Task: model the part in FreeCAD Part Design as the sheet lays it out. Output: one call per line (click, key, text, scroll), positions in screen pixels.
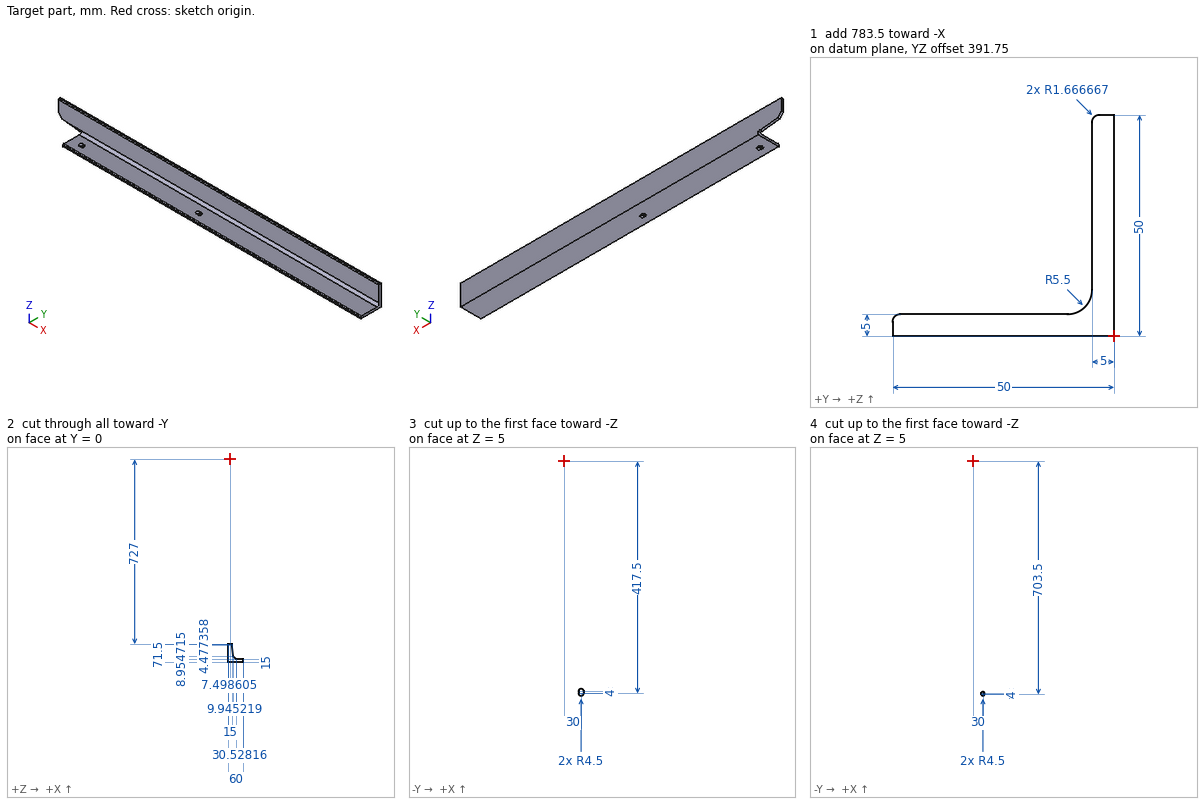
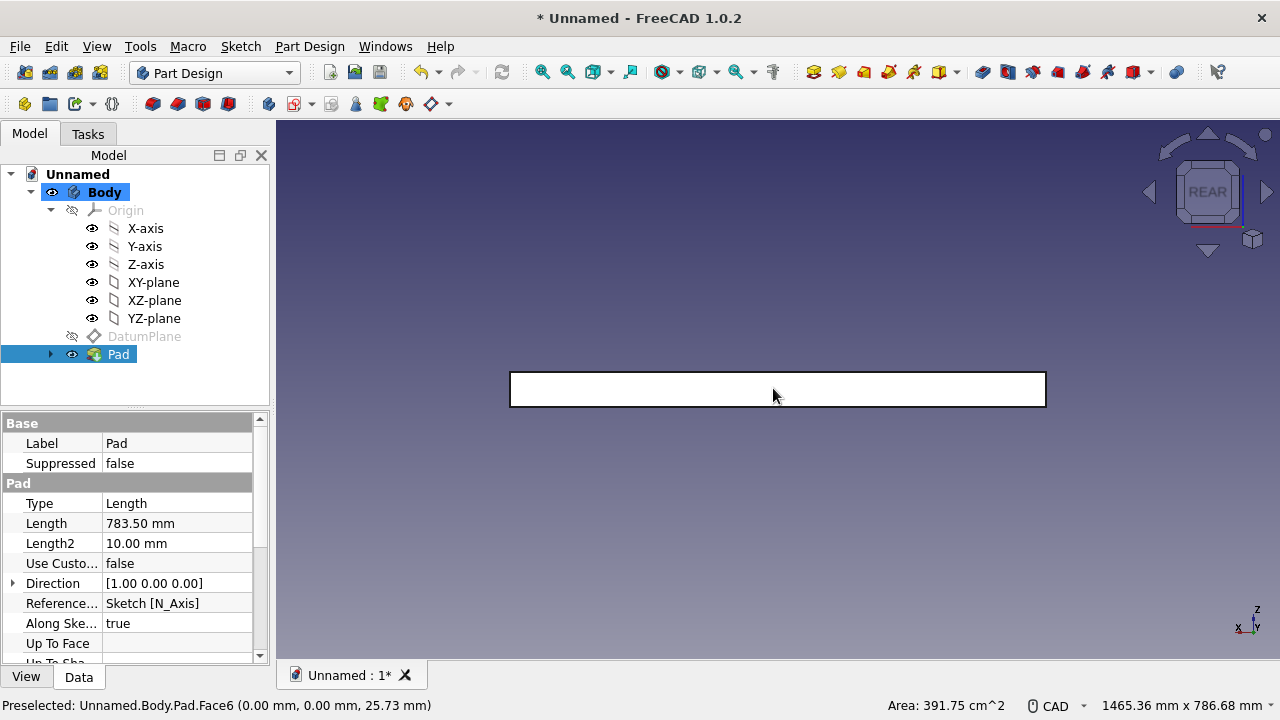
click(294, 104)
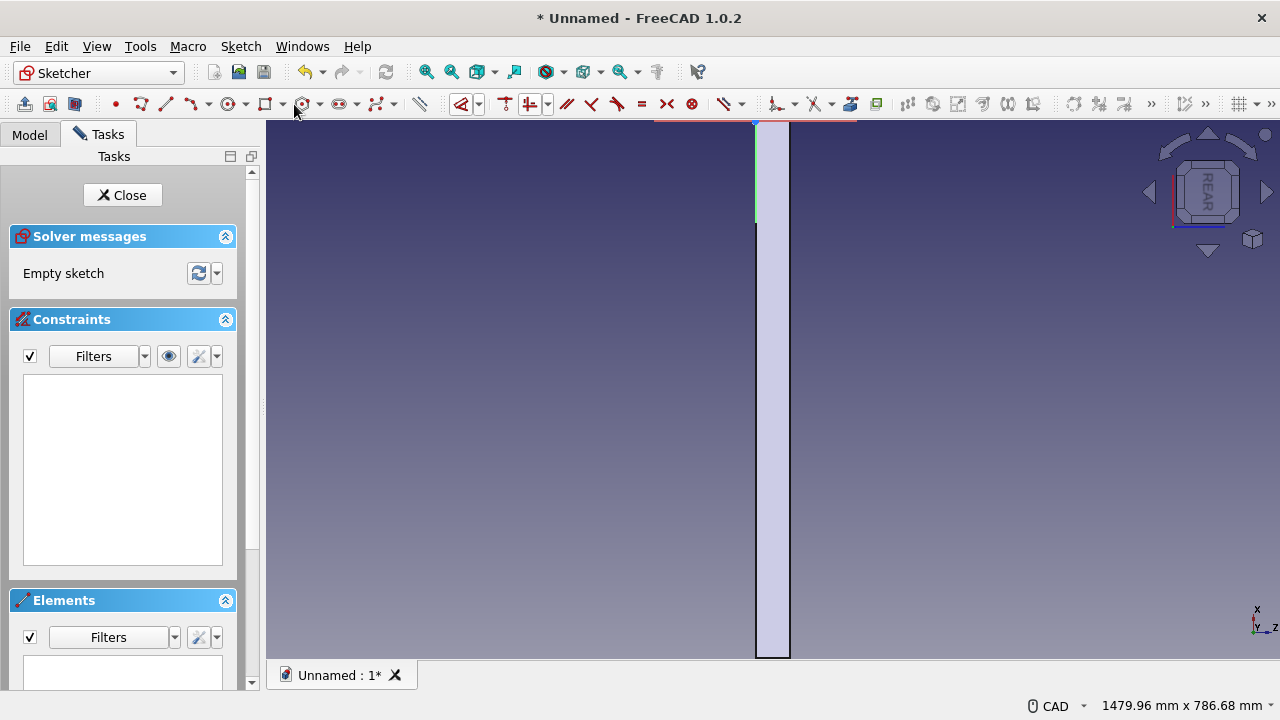
scroll(704, 390, down, 5)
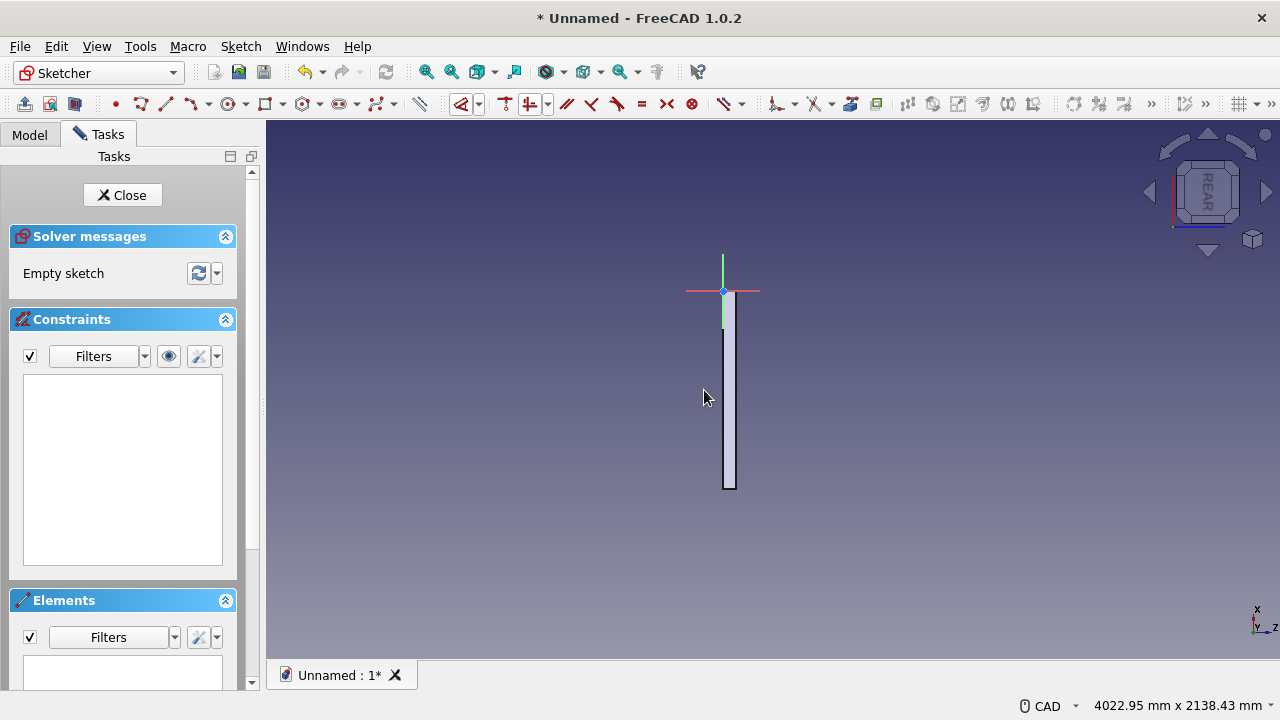
scroll(730, 489, up, 15)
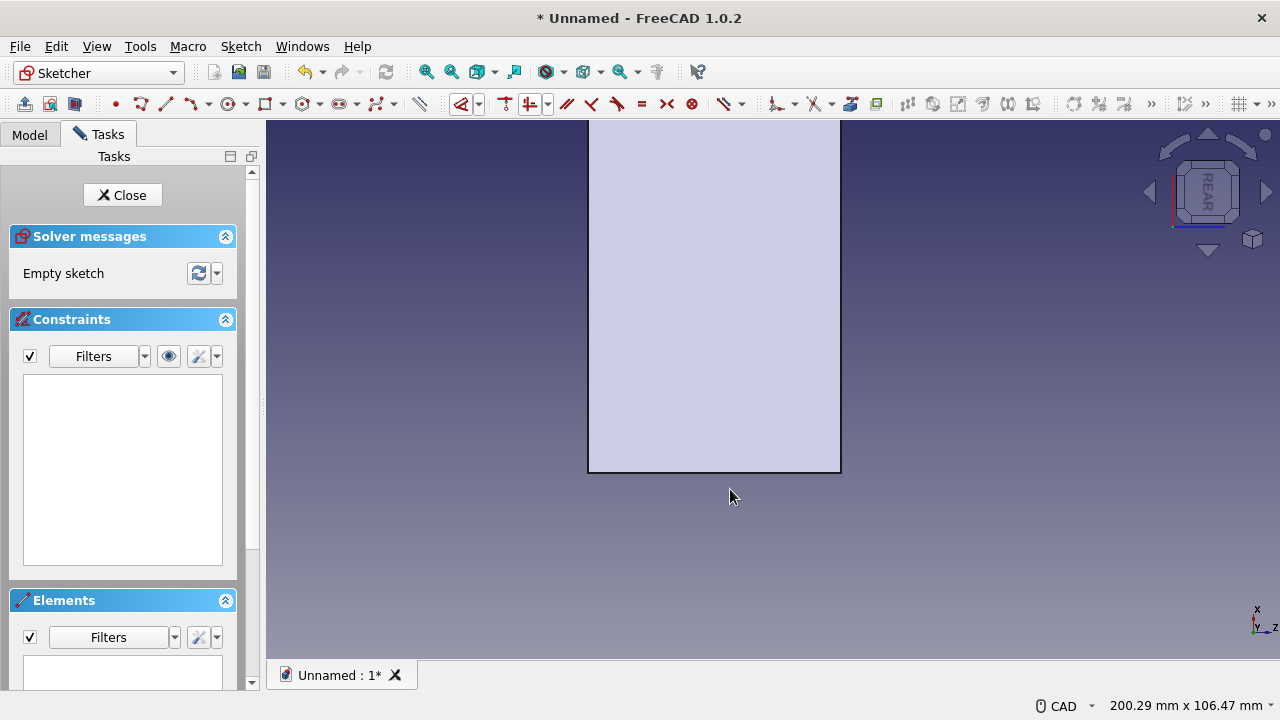
click(141, 104)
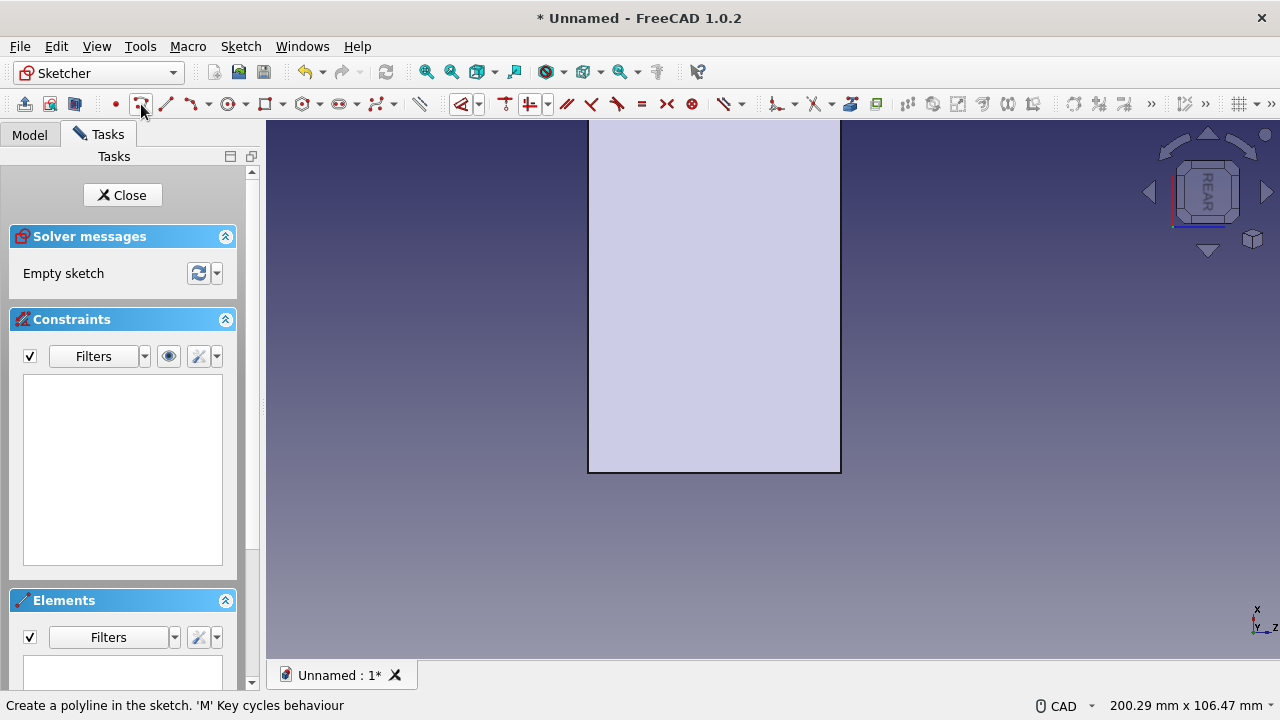
click(550, 187)
click(550, 549)
click(854, 549)
click(854, 473)
click(699, 473)
click(649, 428)
click(626, 210)
click(626, 187)
click(550, 188)
key(Escape)
key(Escape)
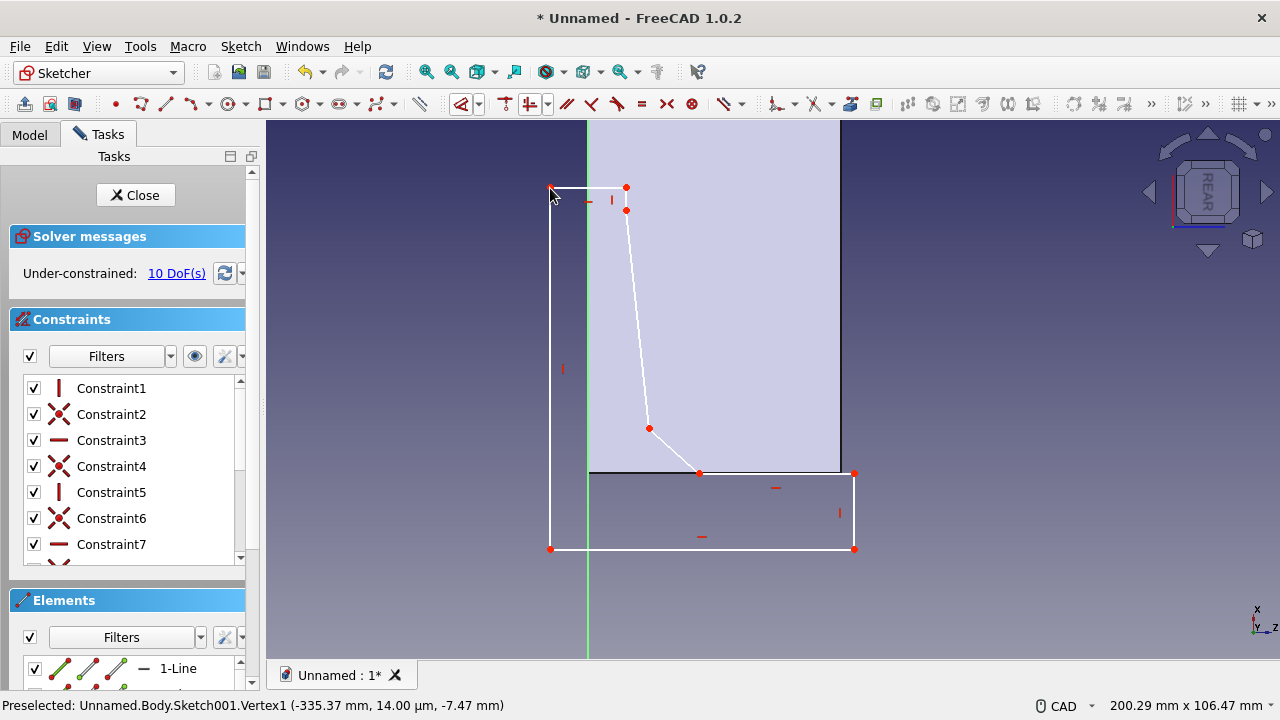
click(641, 550)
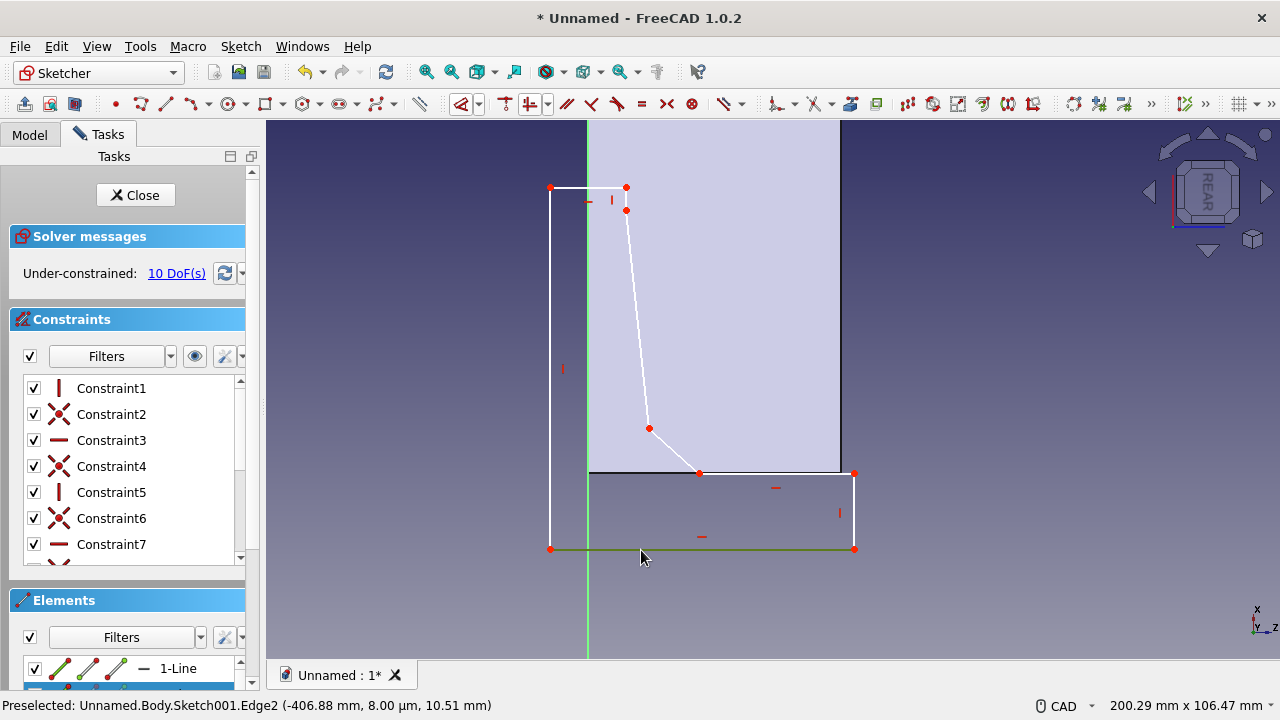
key(l)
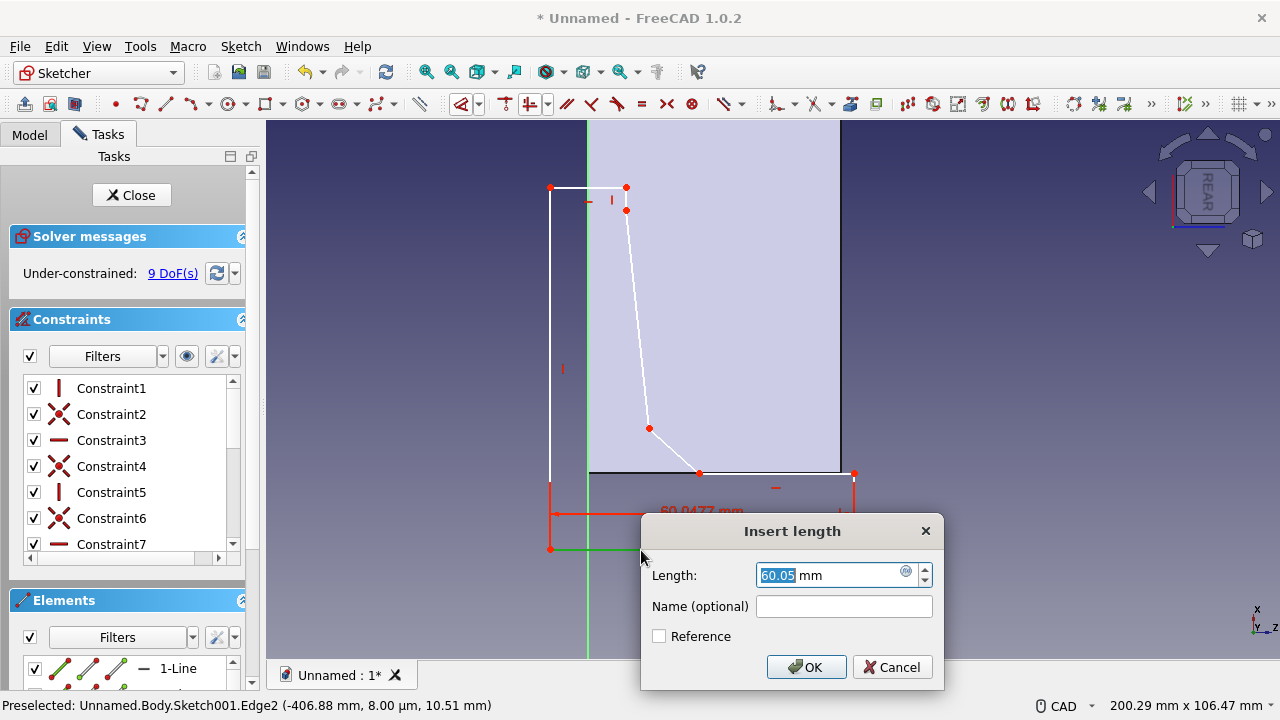
text(60)
key(Return)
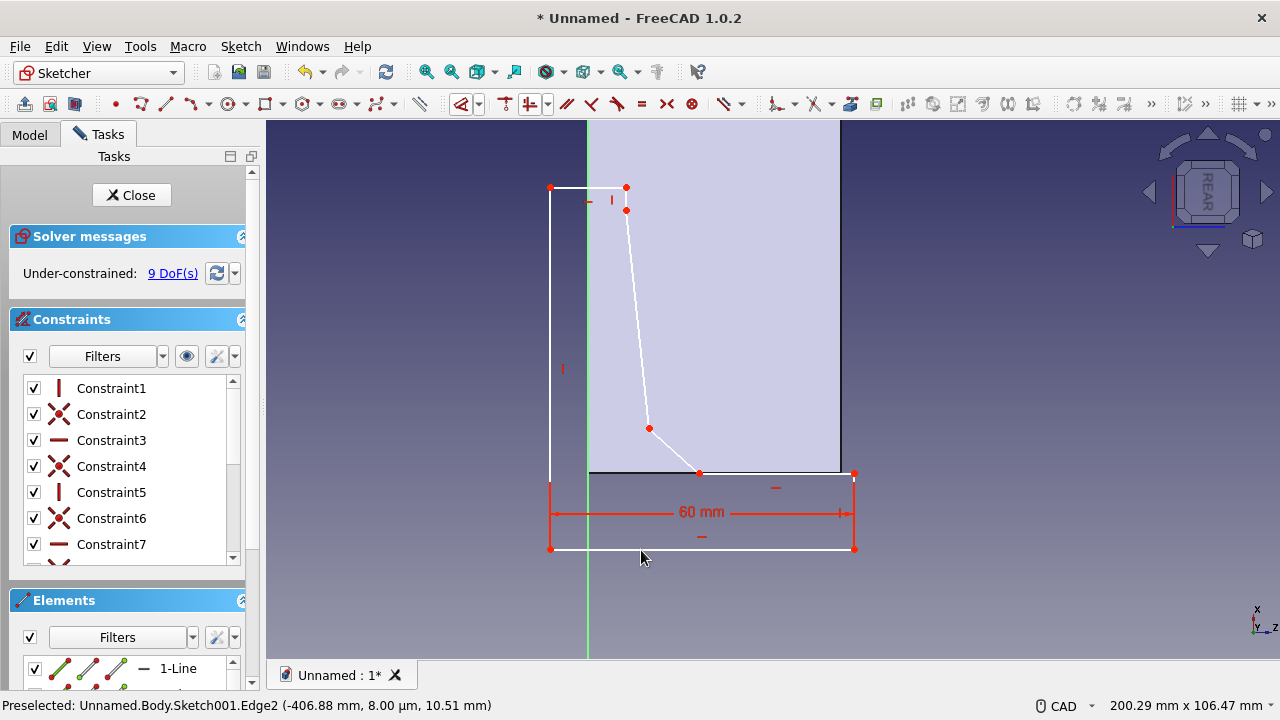
click(854, 527)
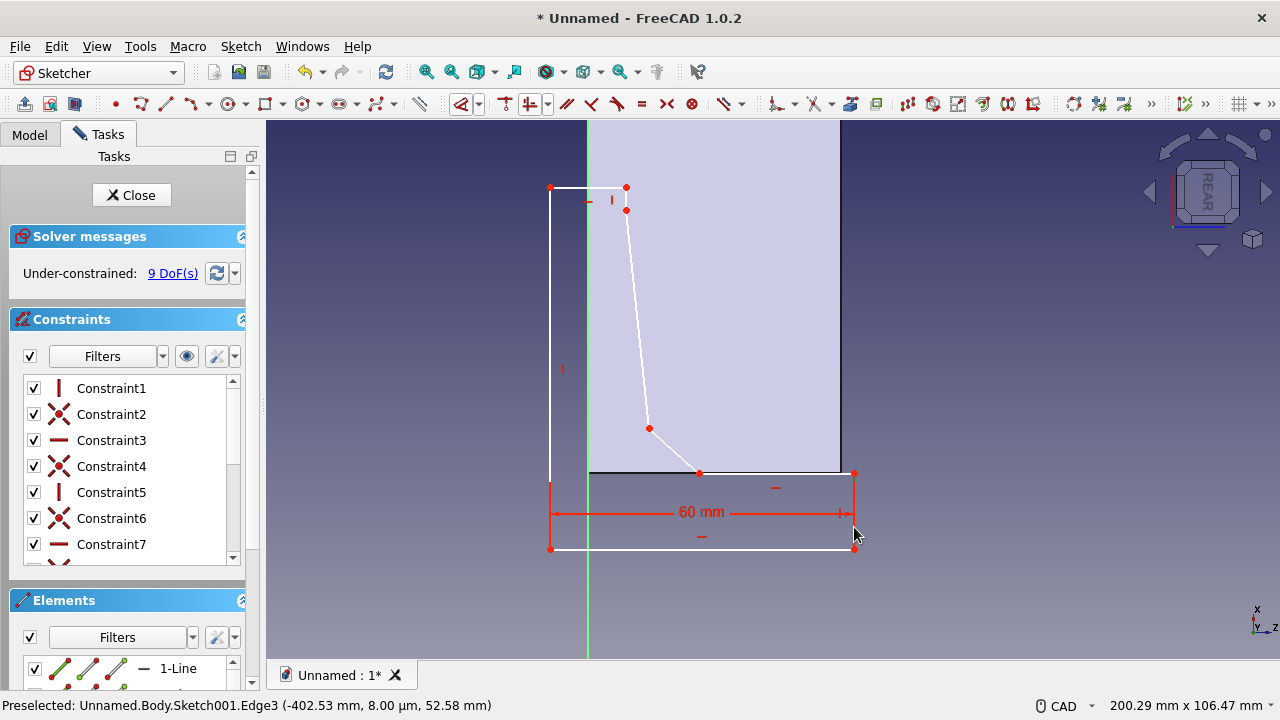
key(i)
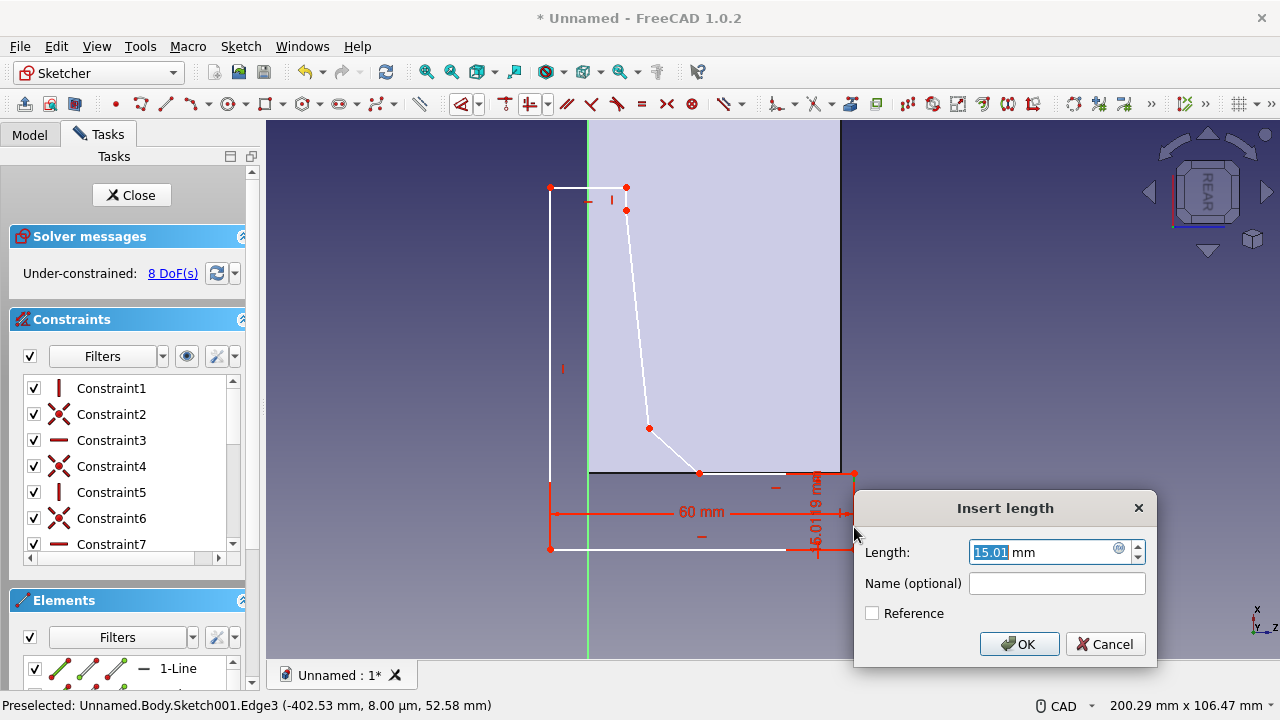
text(15)
key(Return)